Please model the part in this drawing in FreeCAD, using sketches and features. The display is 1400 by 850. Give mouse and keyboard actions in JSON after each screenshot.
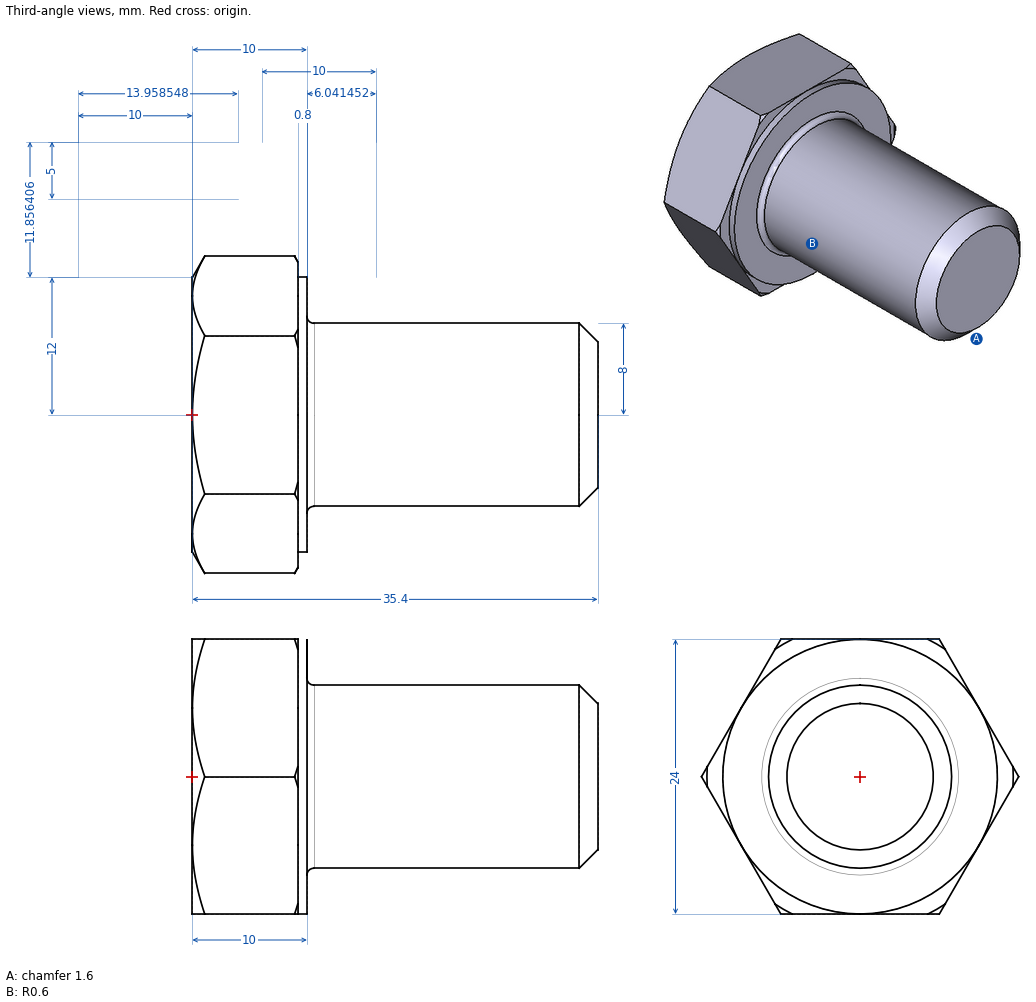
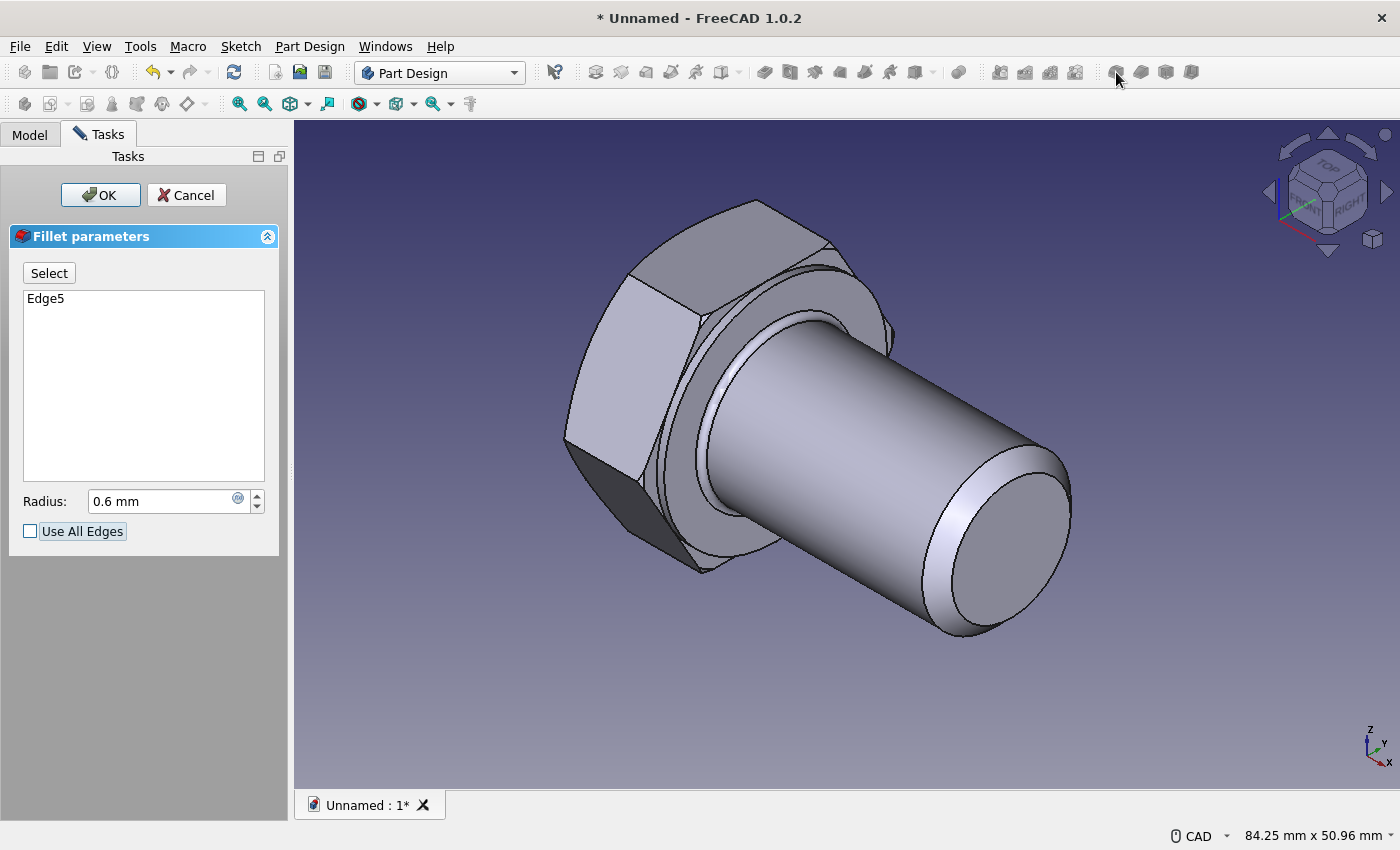
{"action": "left_click", "coordinate": [101, 195]}